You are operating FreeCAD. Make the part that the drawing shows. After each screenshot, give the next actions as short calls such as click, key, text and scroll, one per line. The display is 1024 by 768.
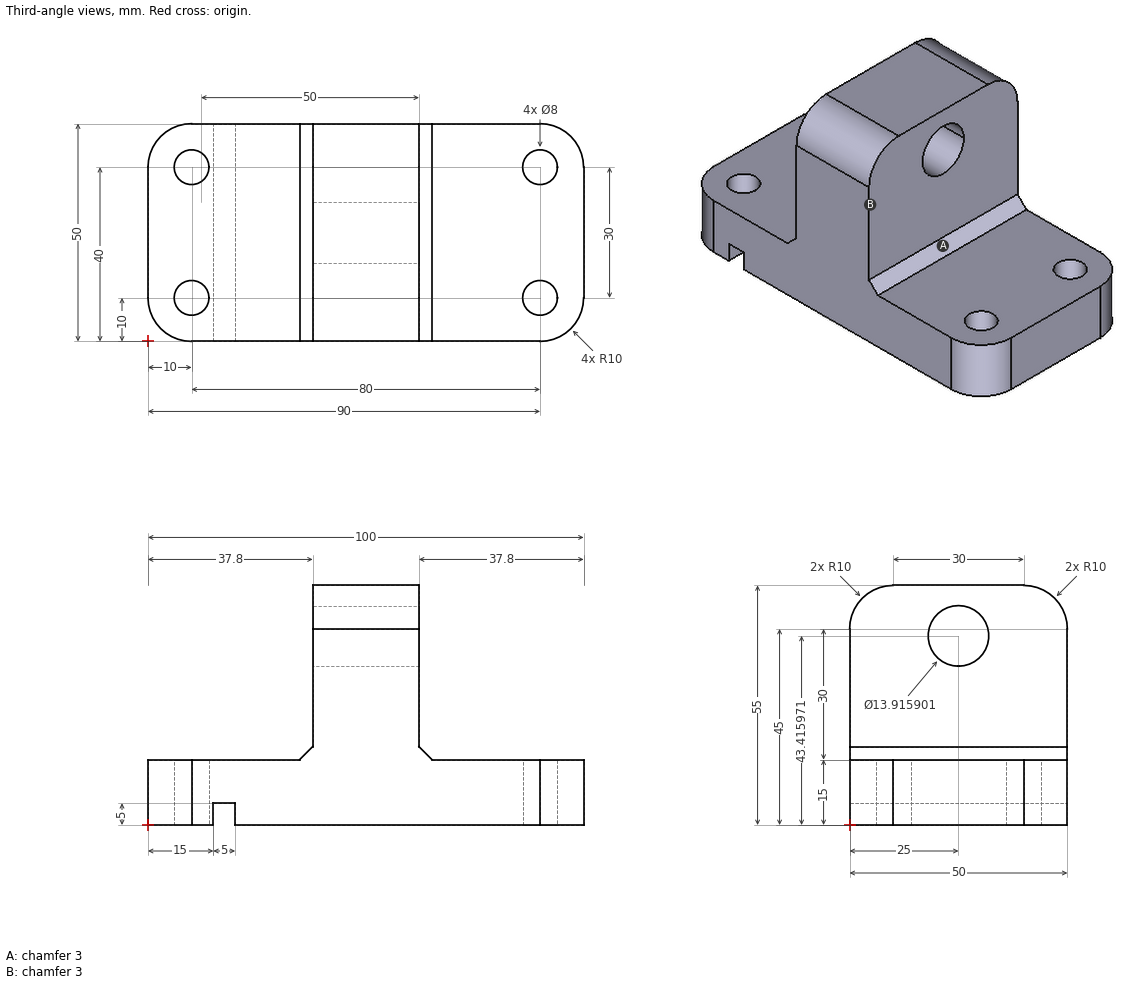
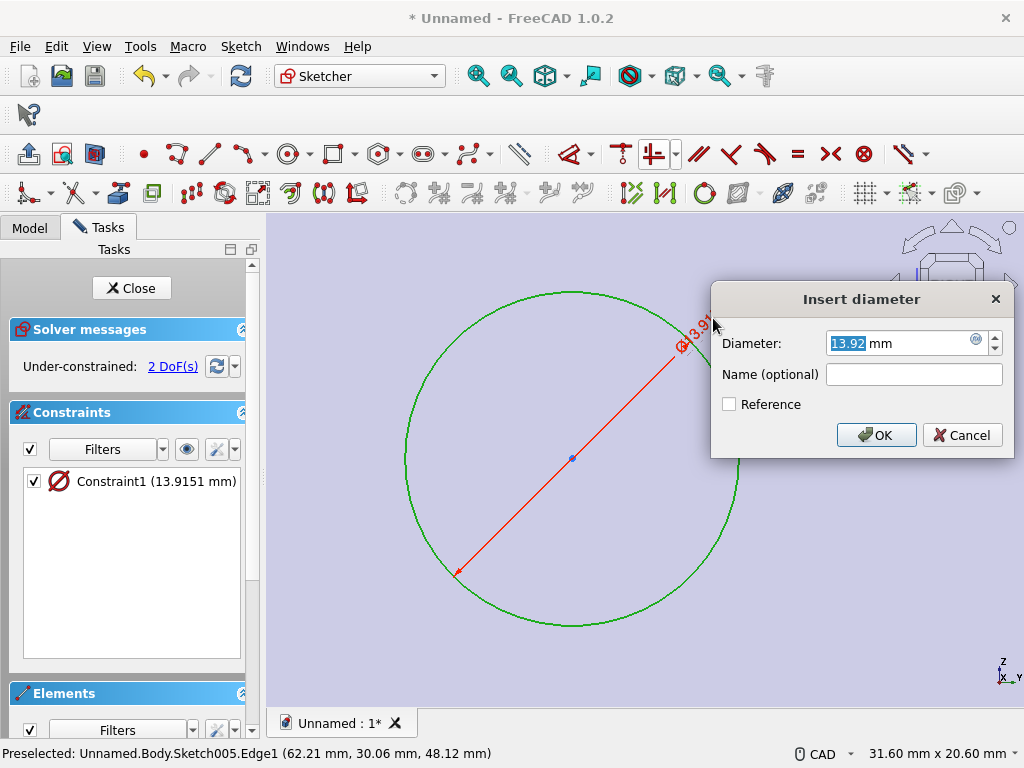
text(13.915901)
key(Return)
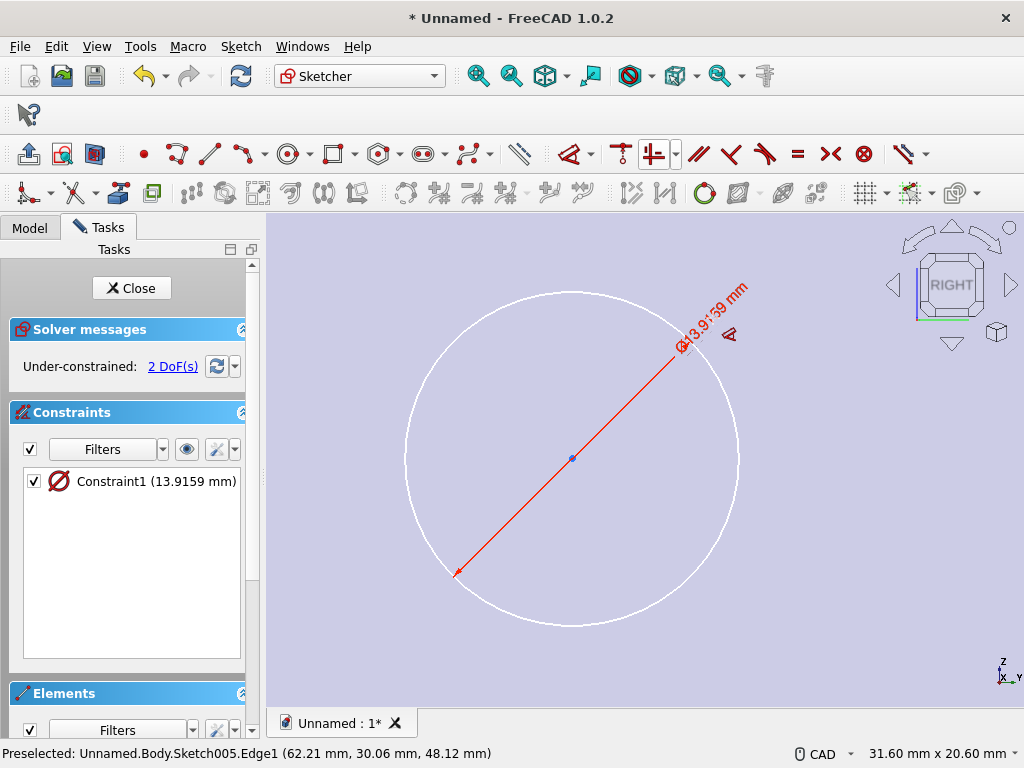
click(572, 459)
click(433, 425)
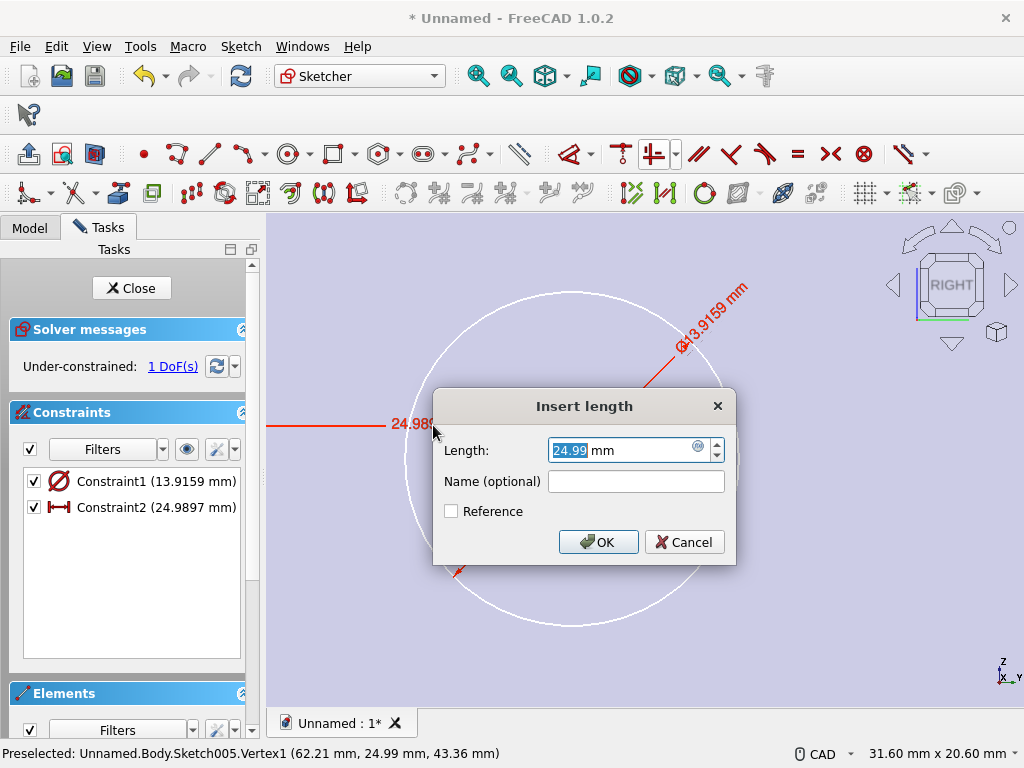
text(25)
key(Return)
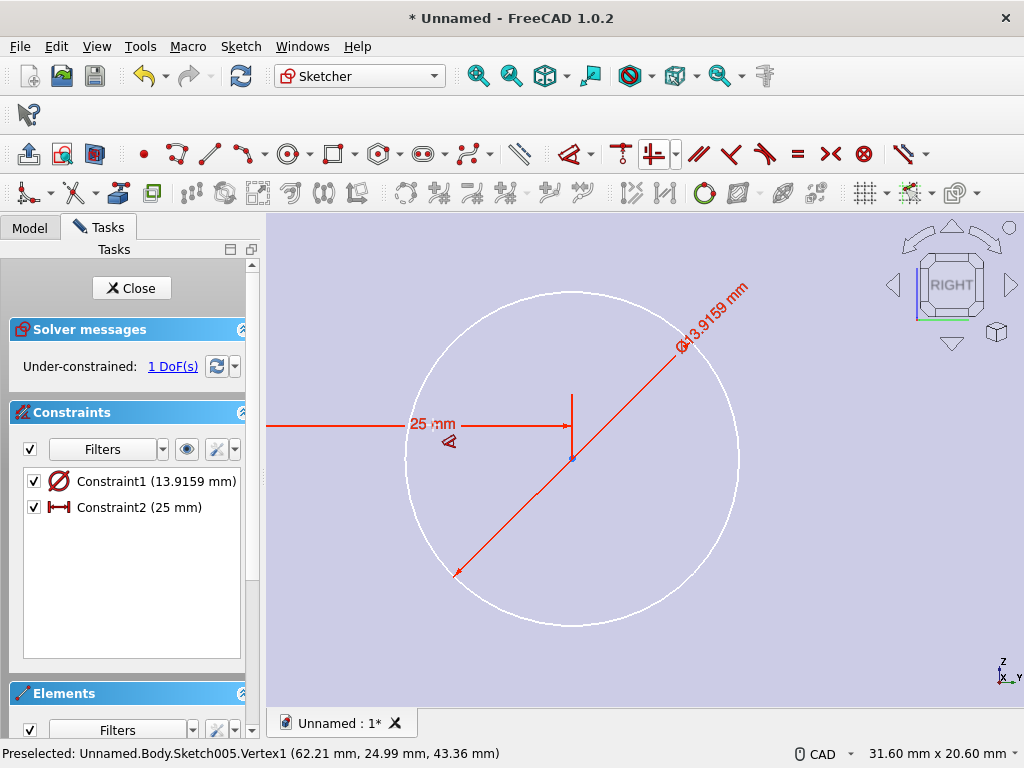
click(572, 459)
click(606, 569)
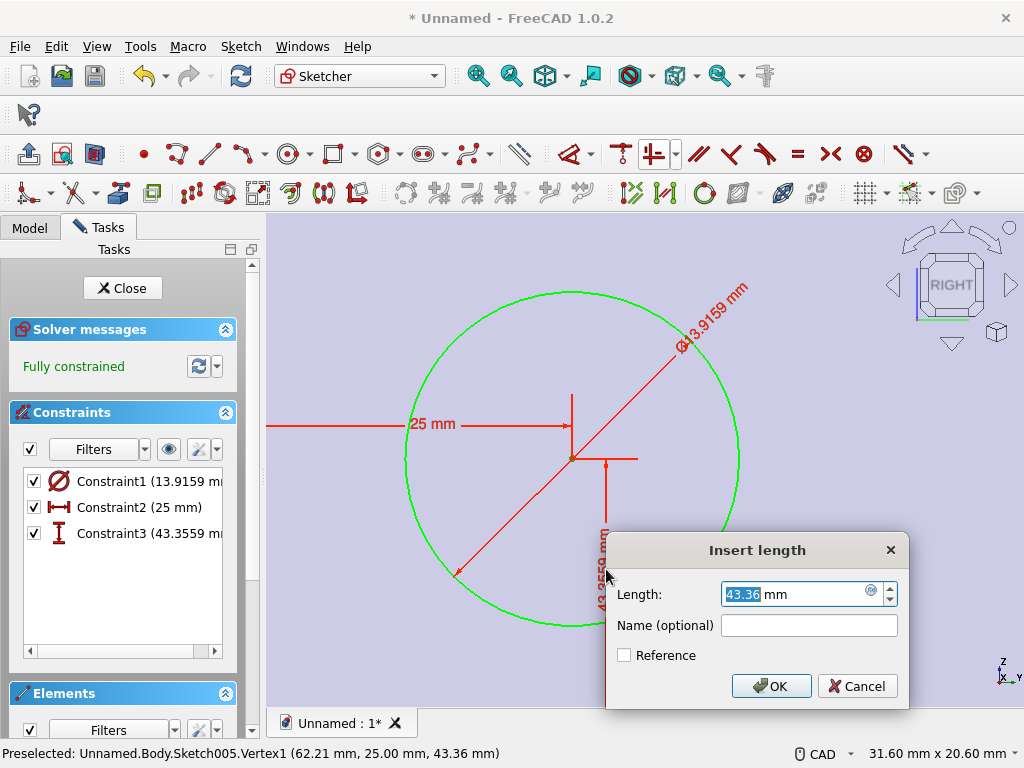
text(43.415971)
key(Return)
key(Escape)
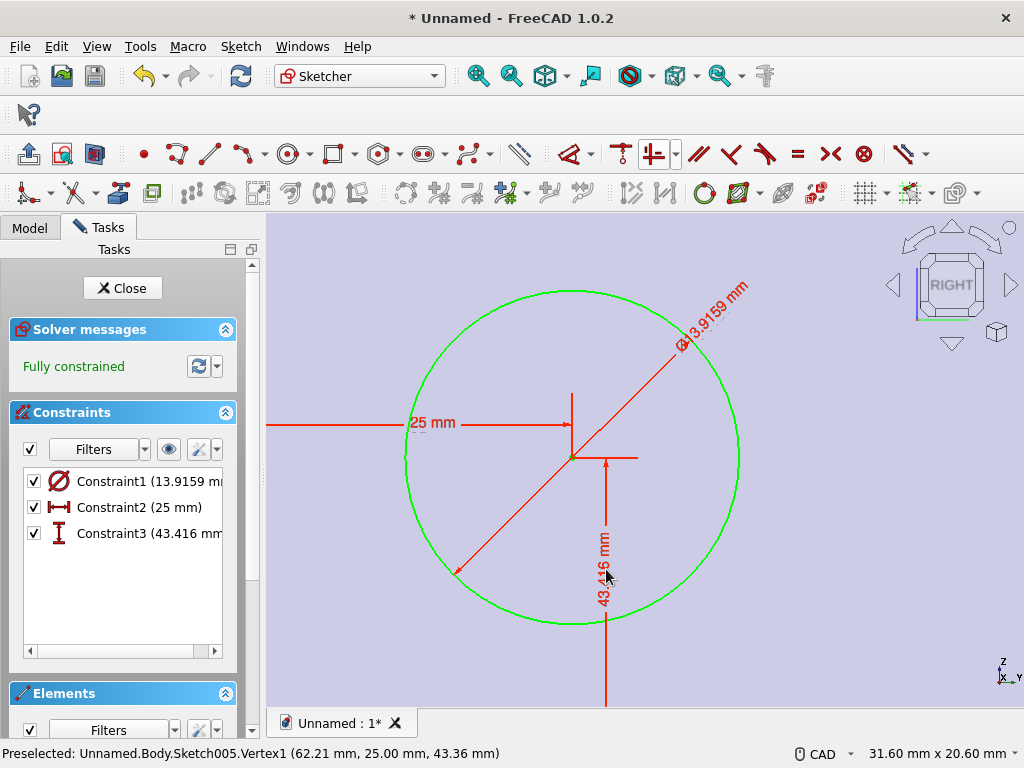
click(123, 288)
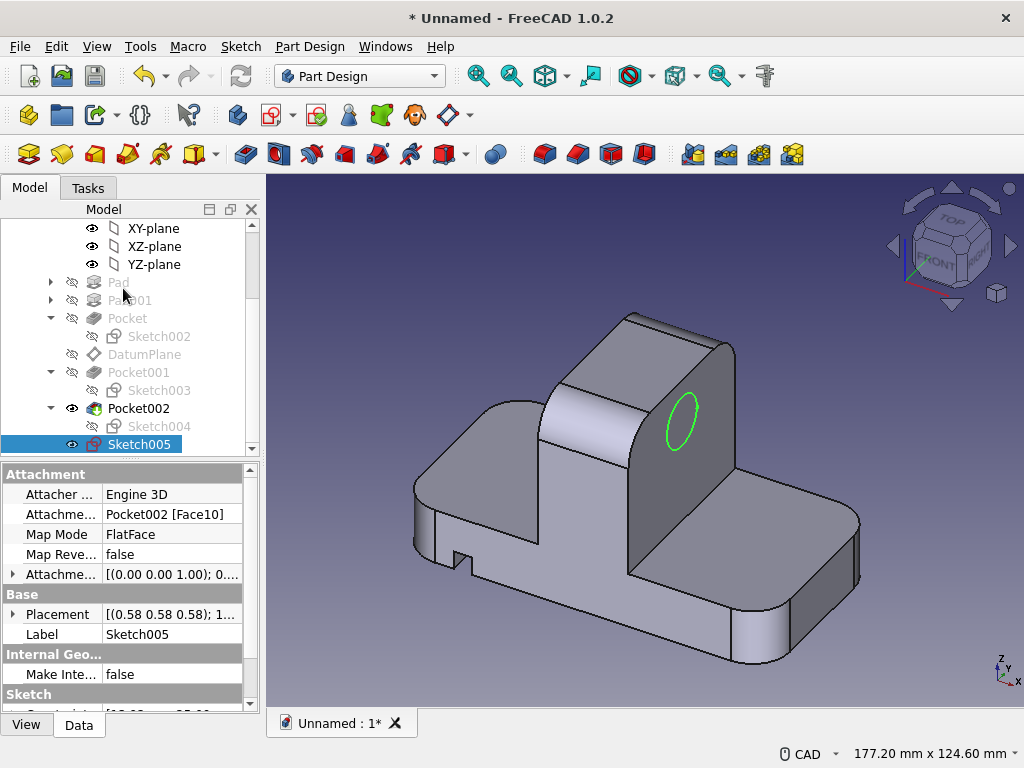
click(246, 154)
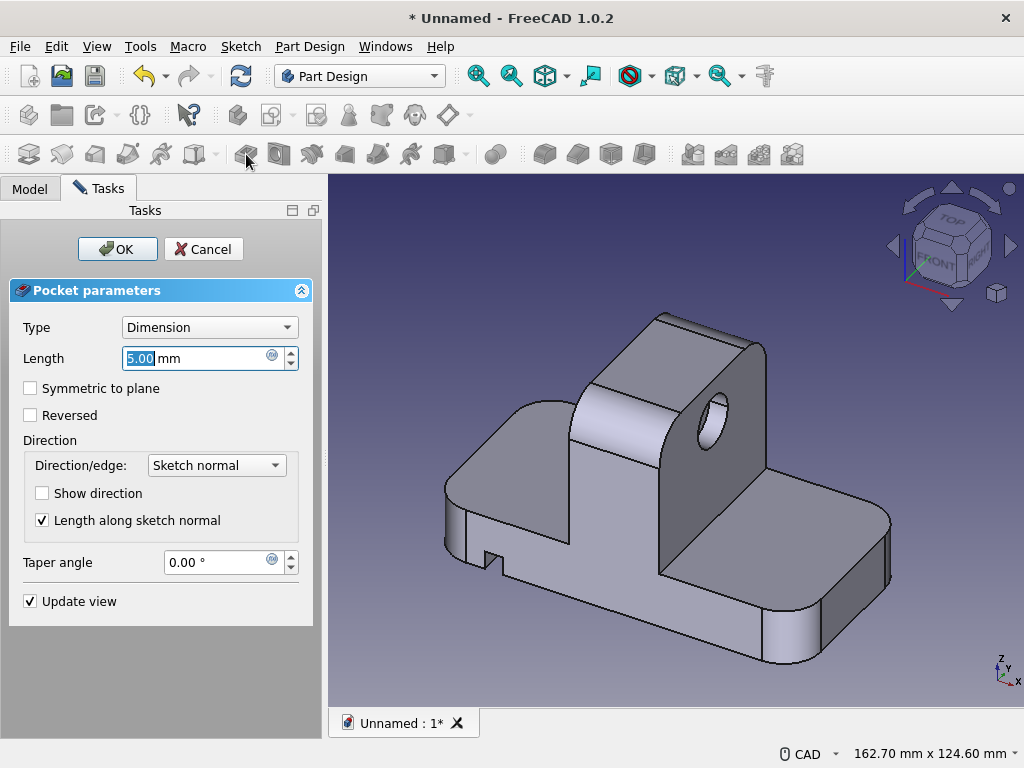
text(50)
key(Tab)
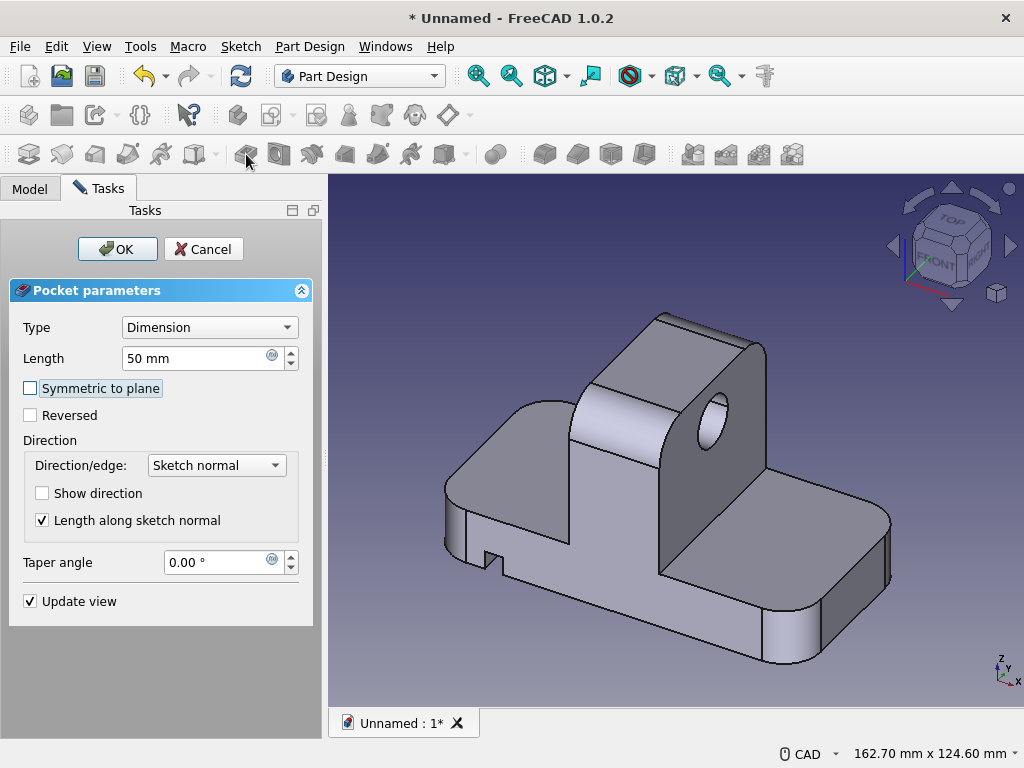
click(118, 249)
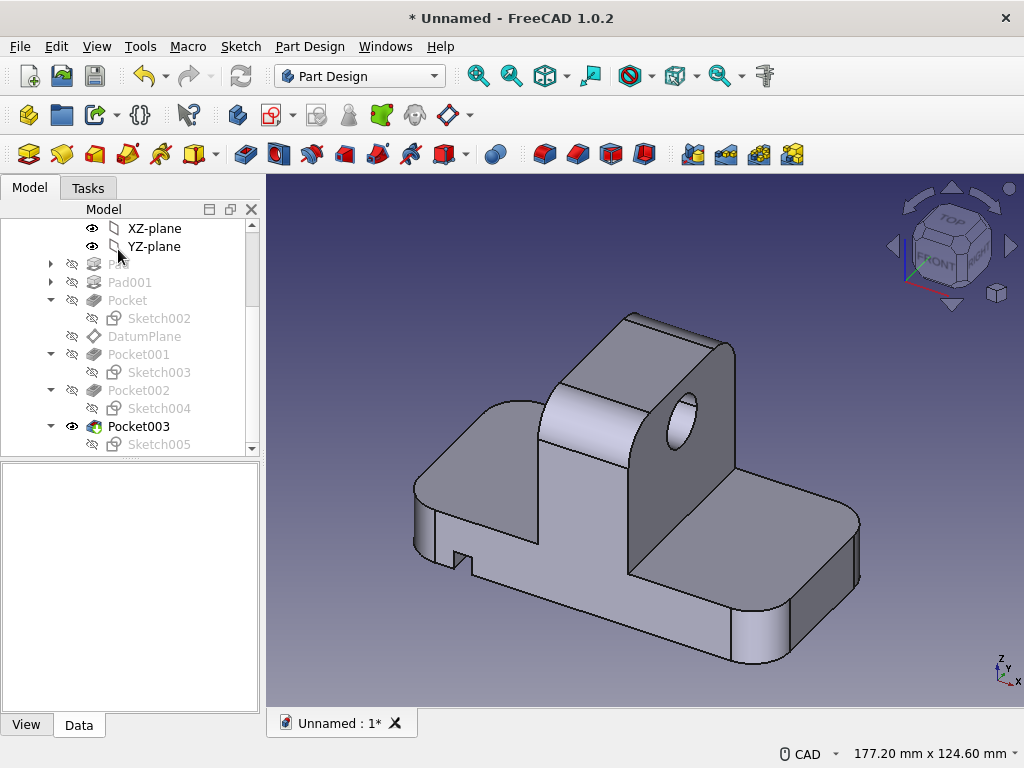
click(752, 543)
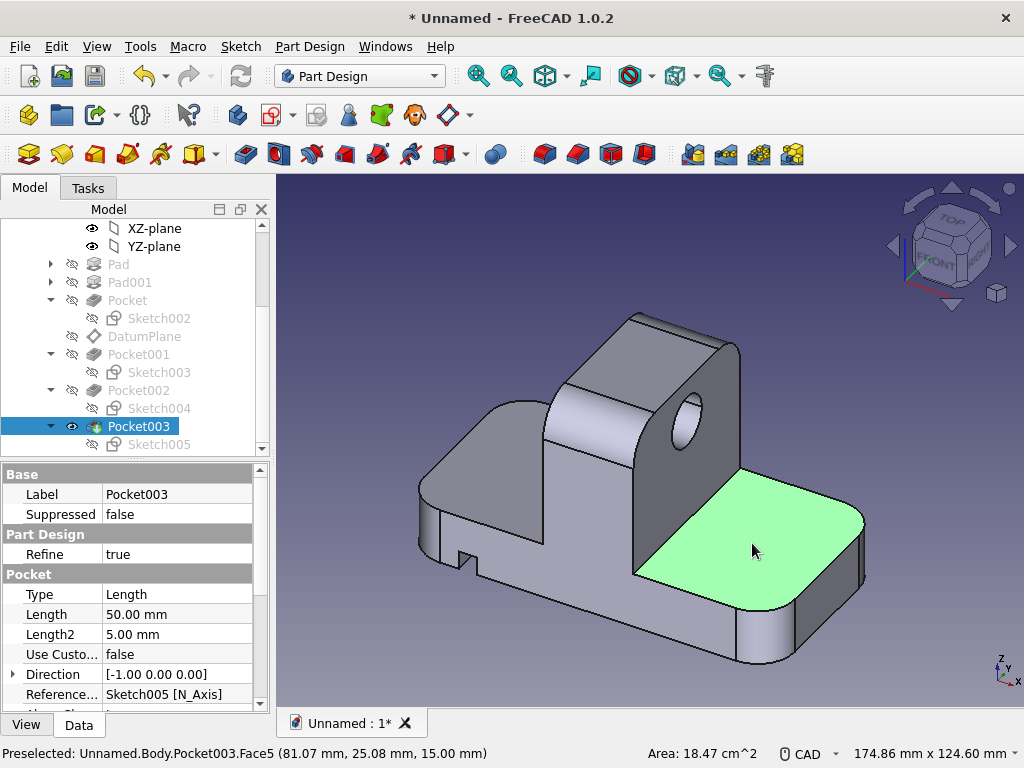
click(270, 116)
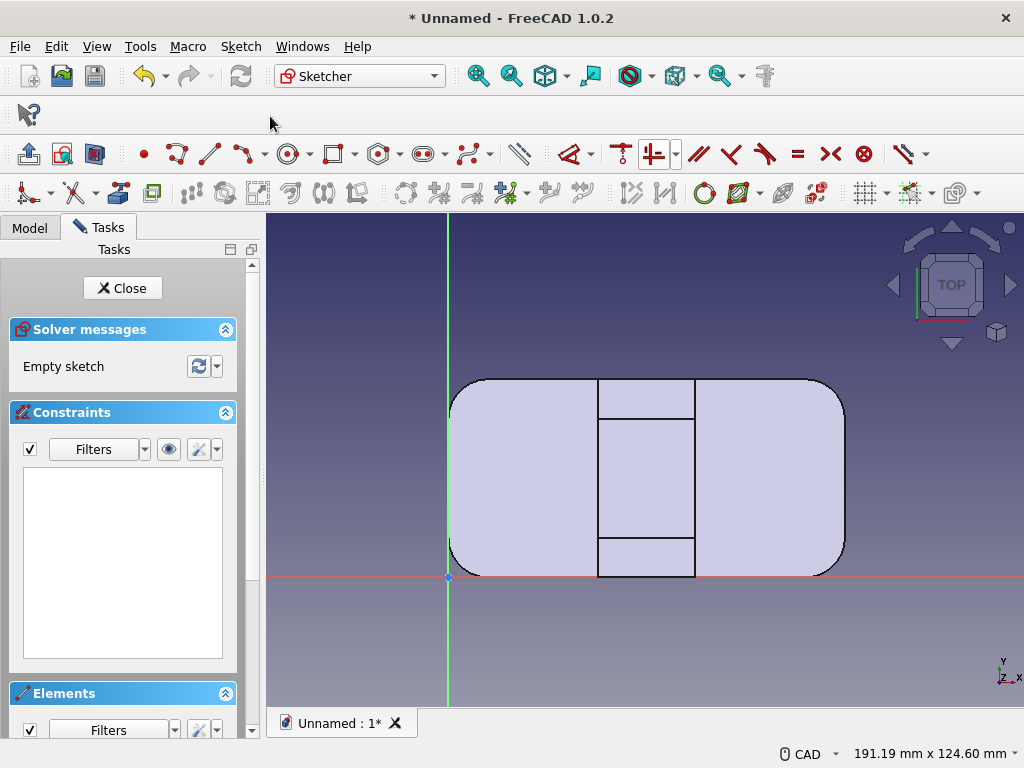
click(95, 154)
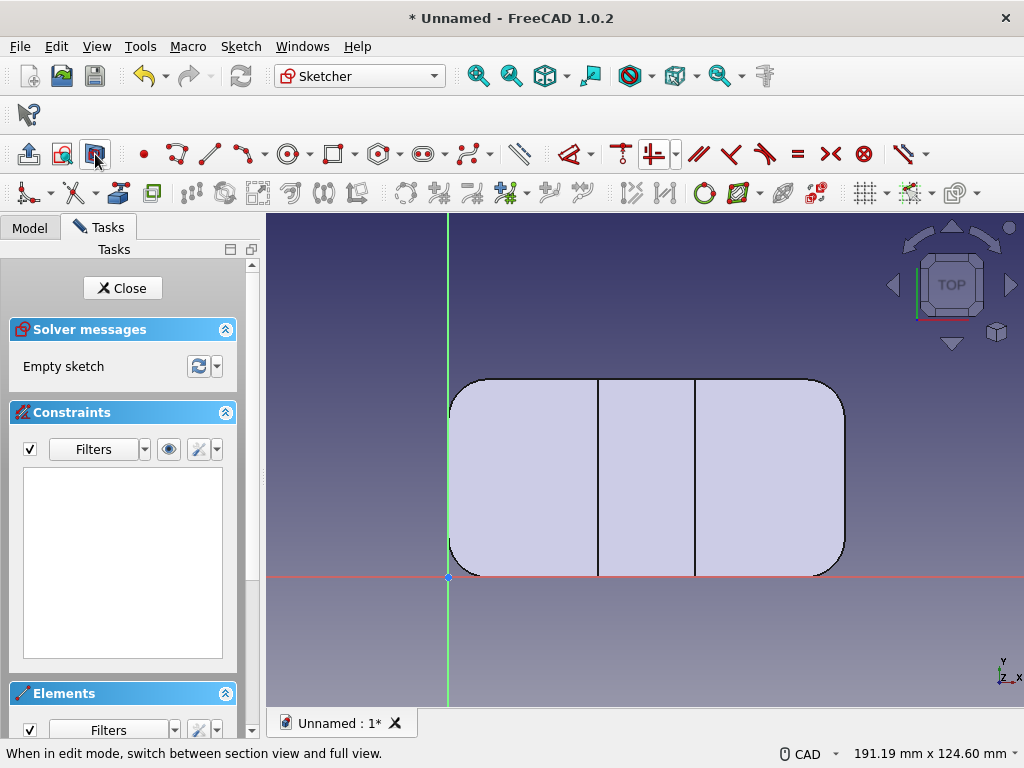
click(288, 154)